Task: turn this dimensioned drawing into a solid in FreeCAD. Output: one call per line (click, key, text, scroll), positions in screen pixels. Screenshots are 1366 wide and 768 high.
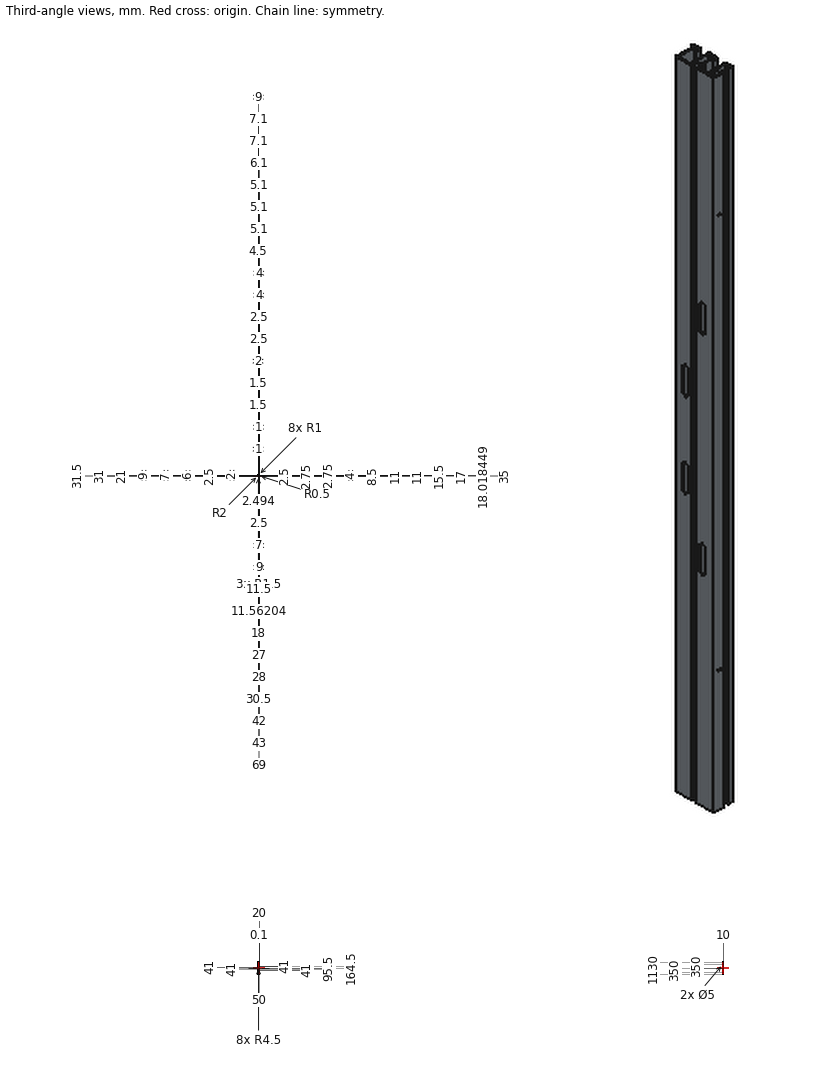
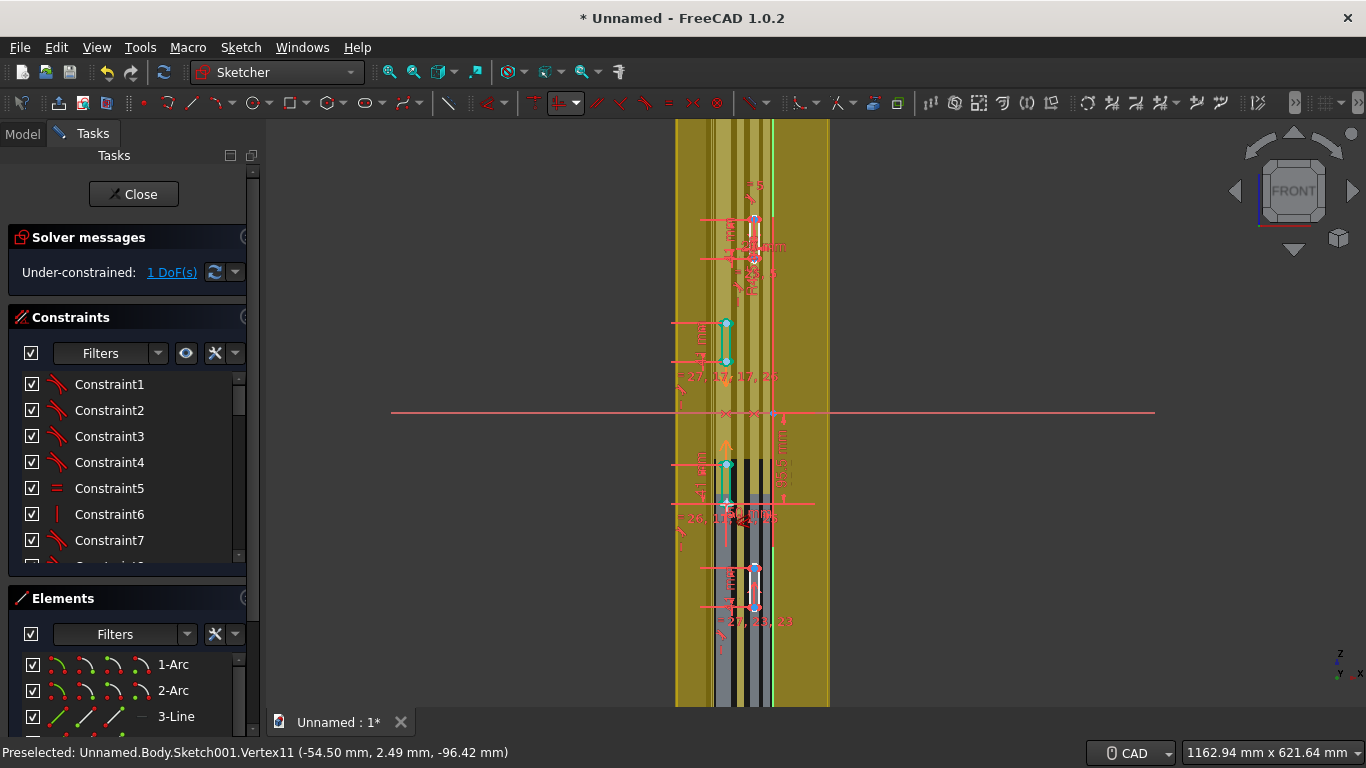
scroll(750, 259, up, 6)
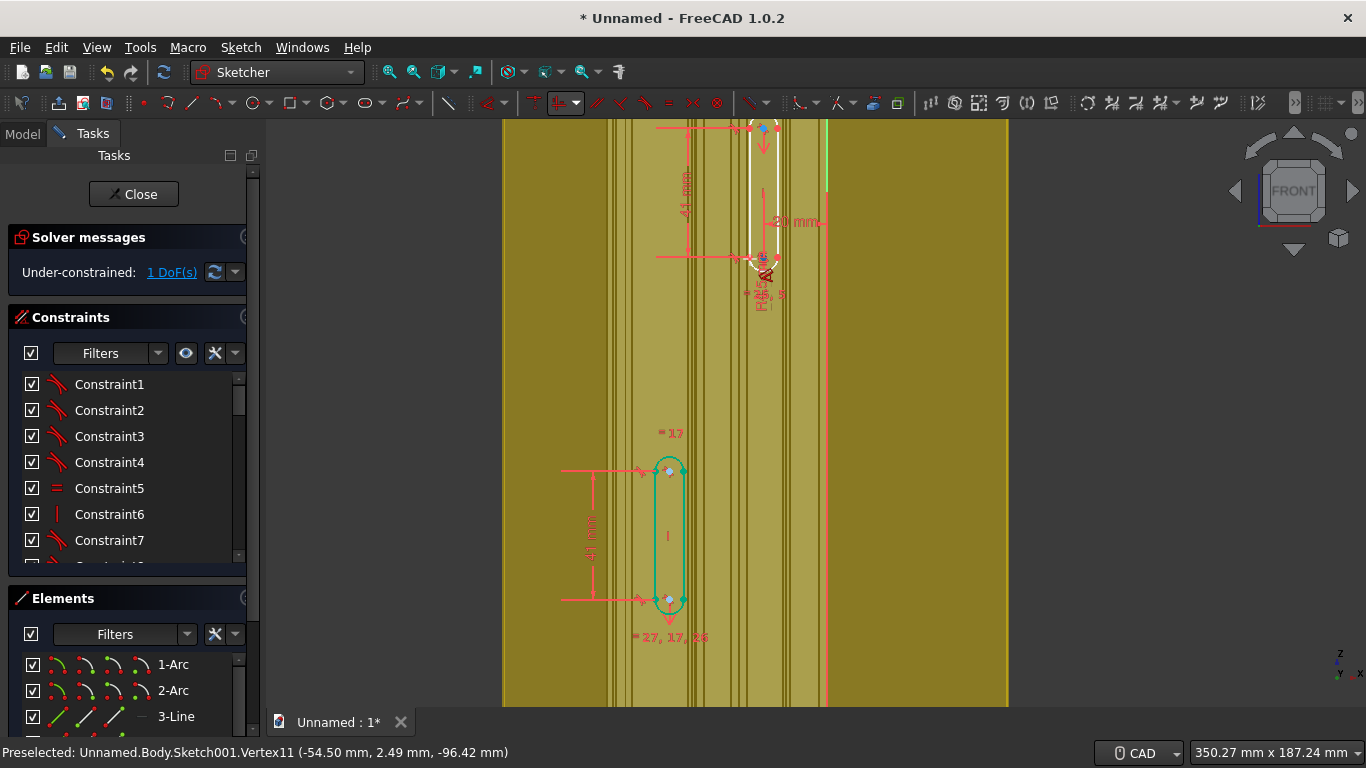
click(750, 257)
click(861, 468)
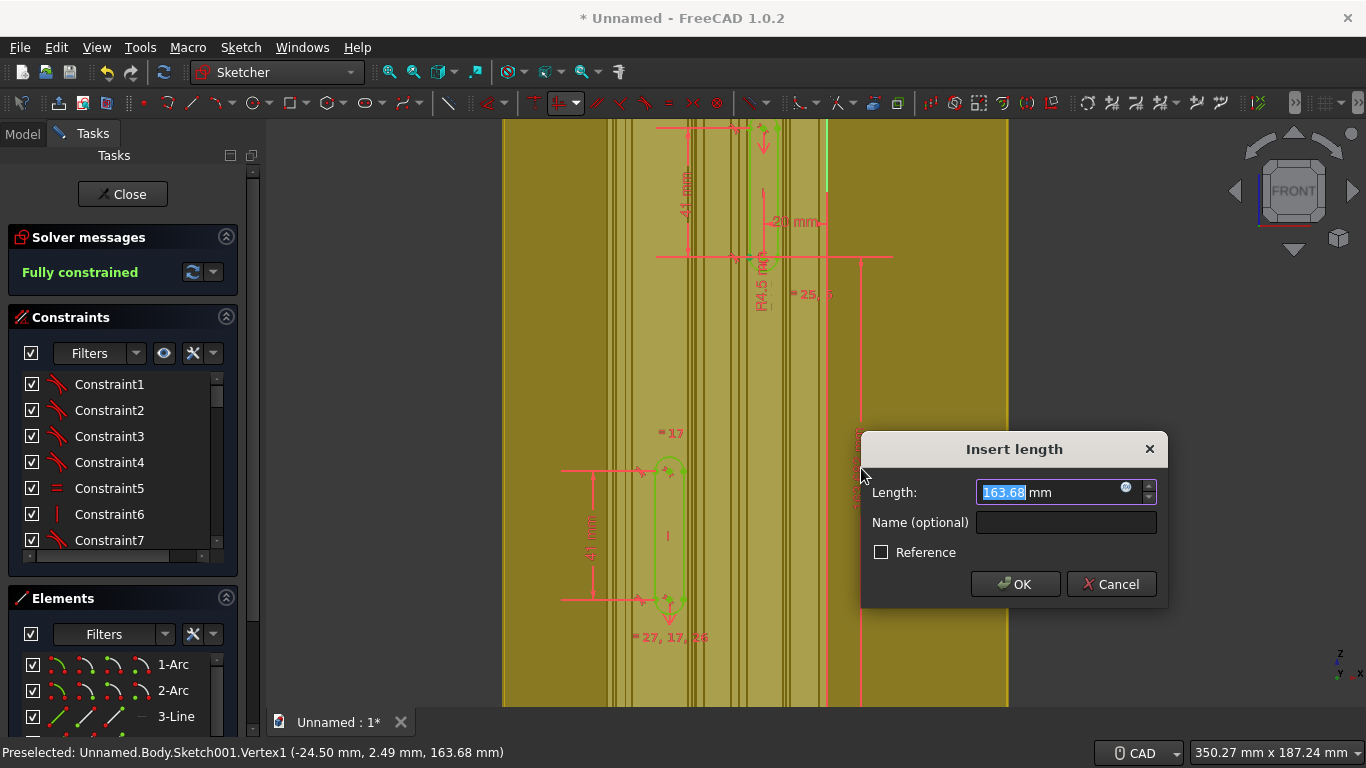
text(164.5)
key(Return)
key(Escape)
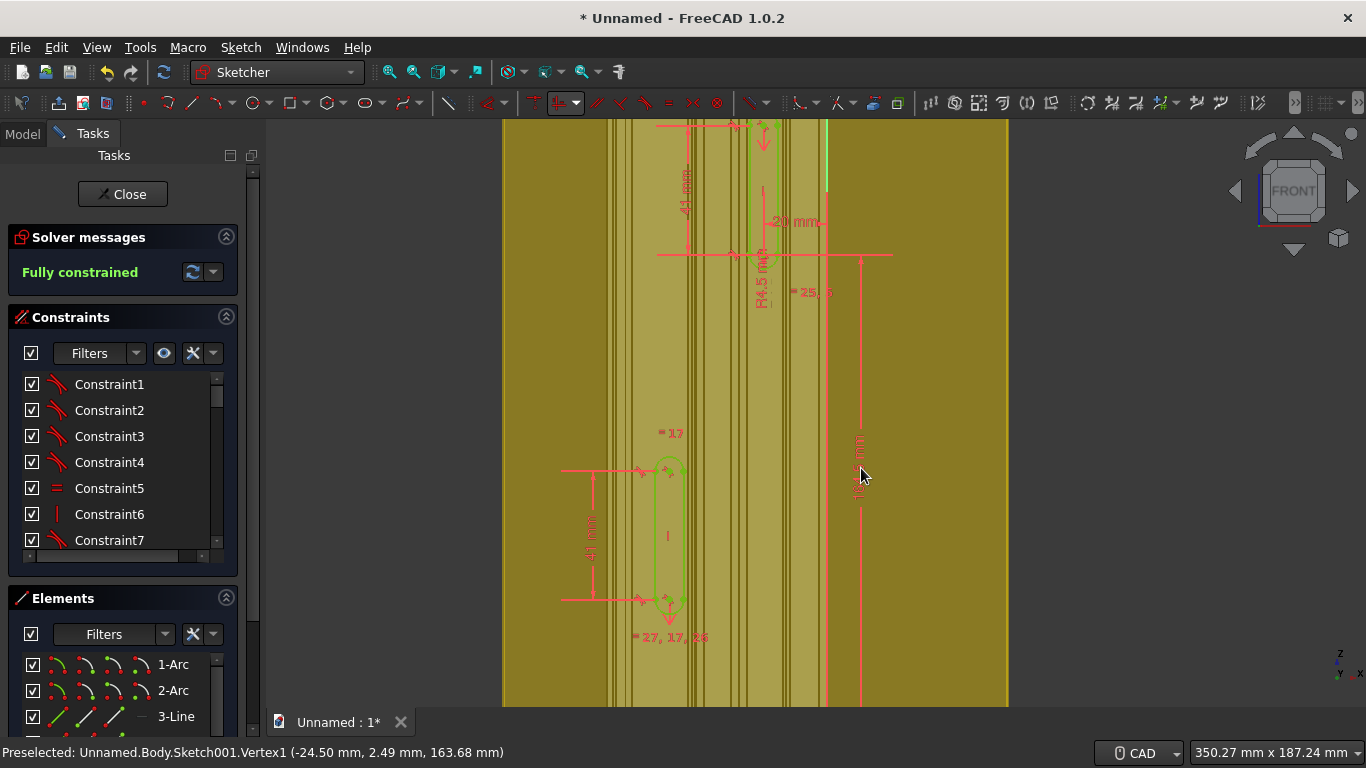
click(123, 194)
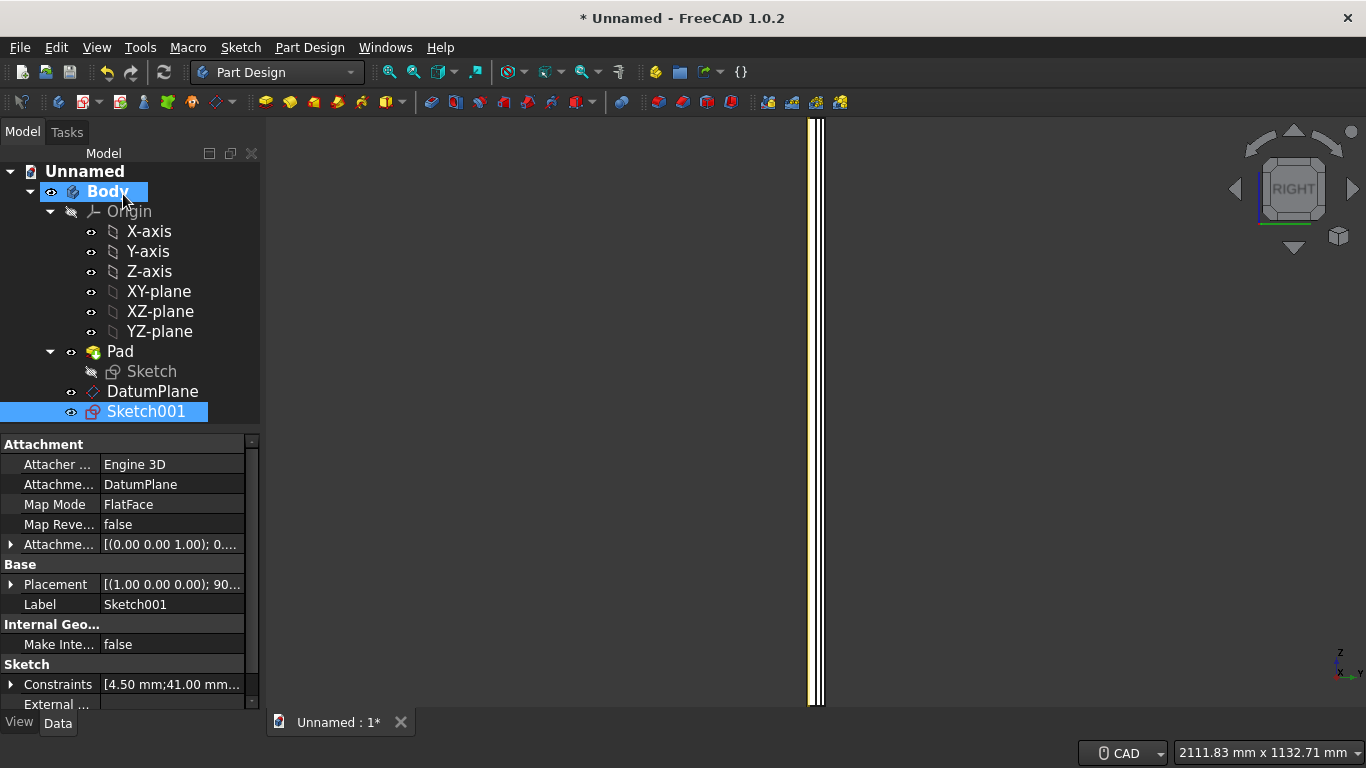
click(432, 102)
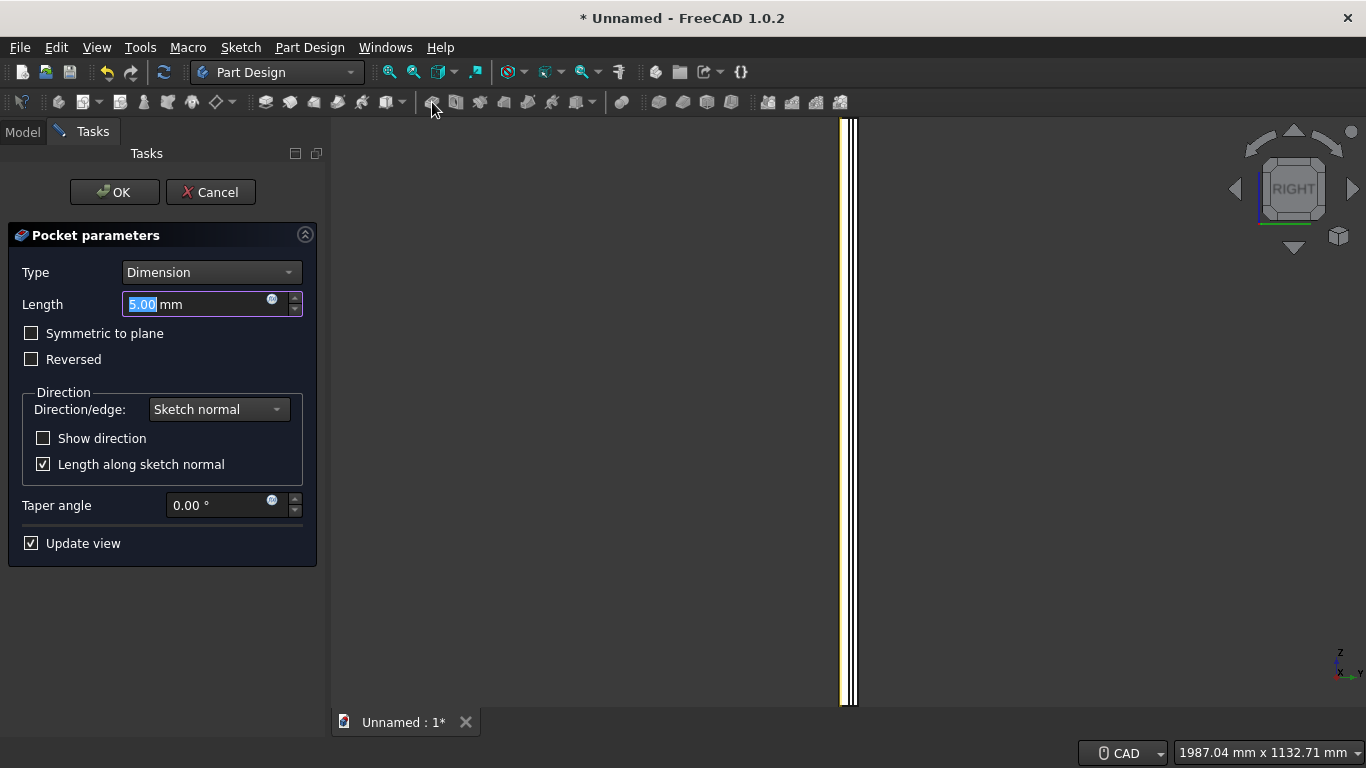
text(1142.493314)
key(Tab)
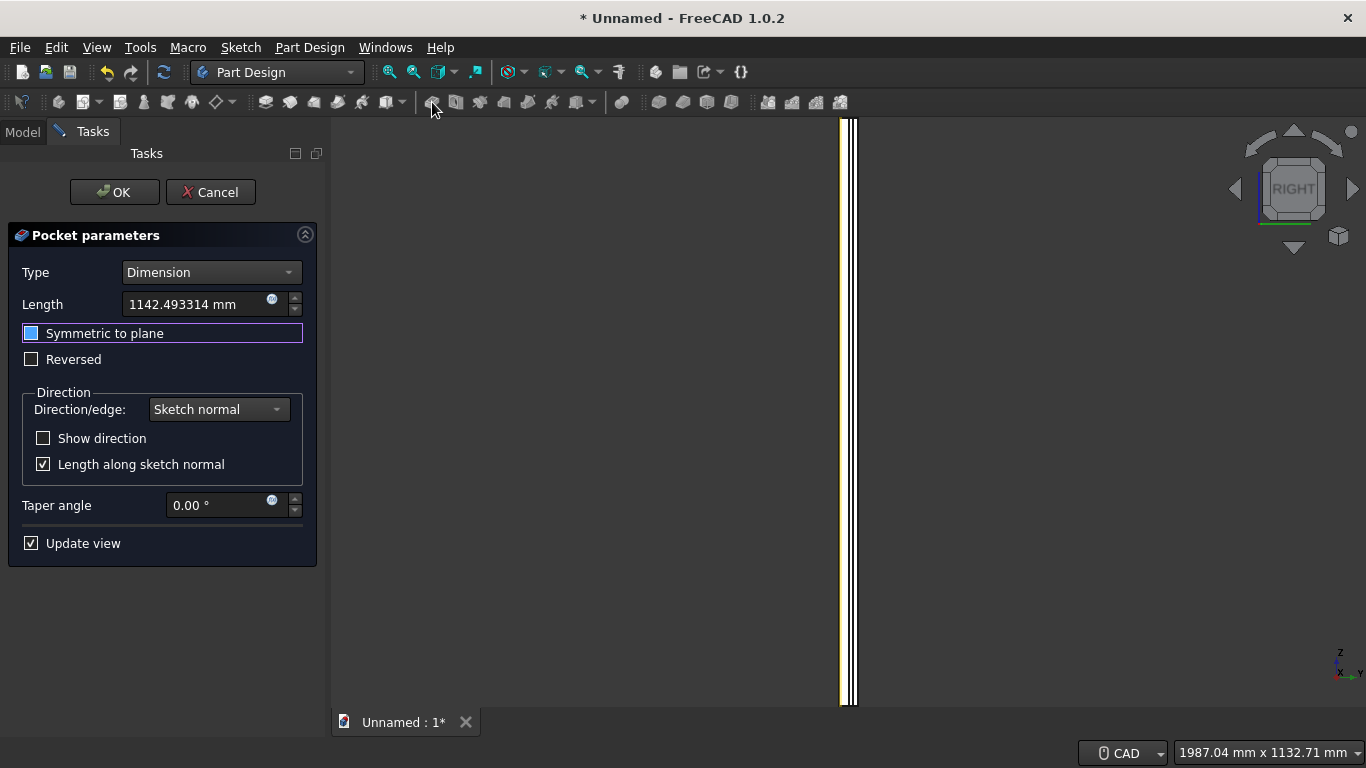
click(30, 333)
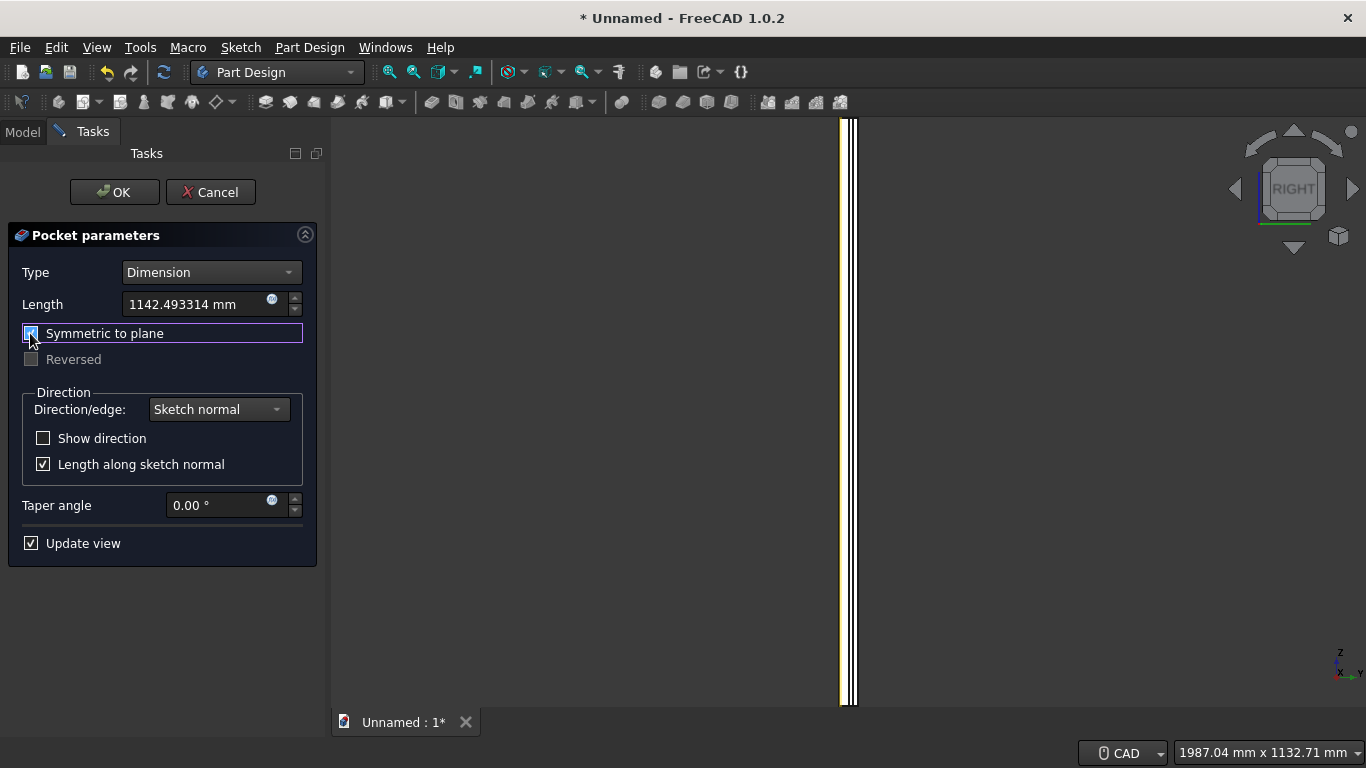
click(115, 192)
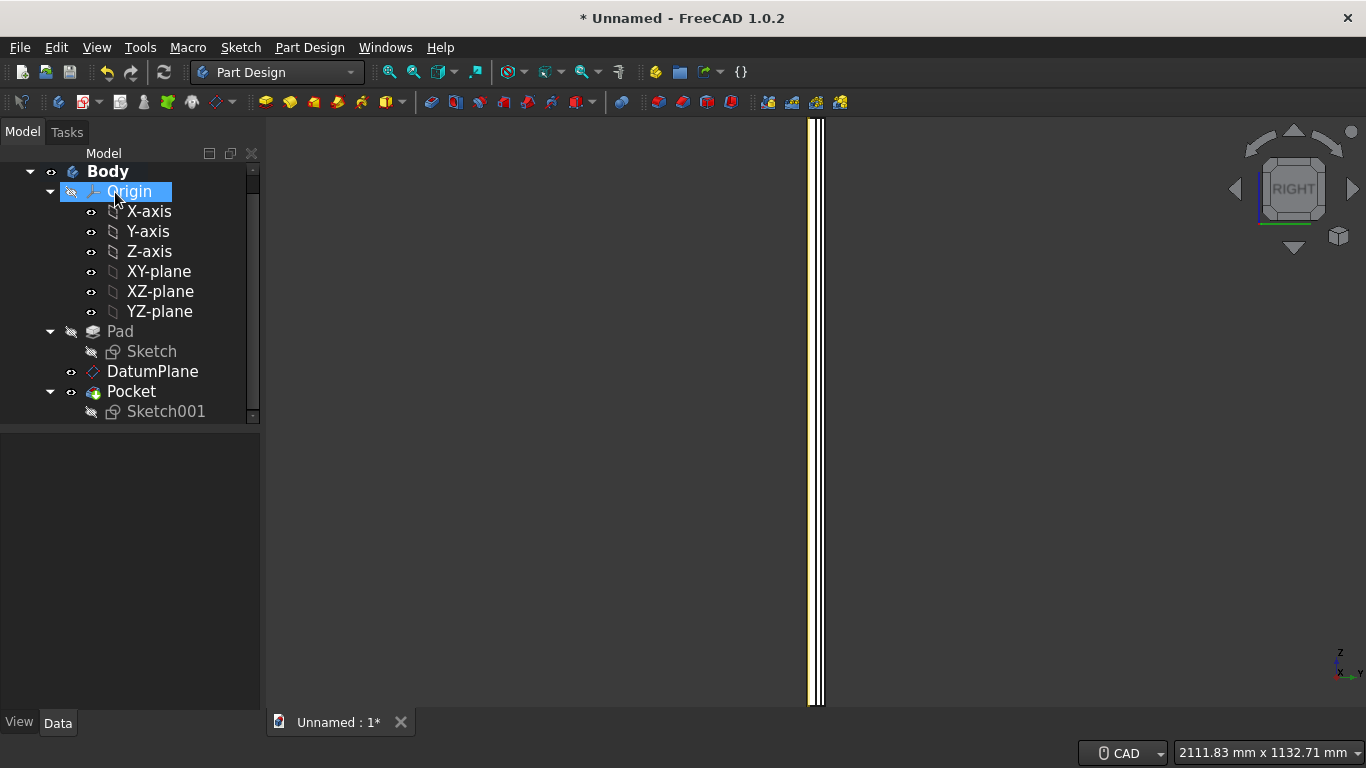
click(116, 372)
key(space)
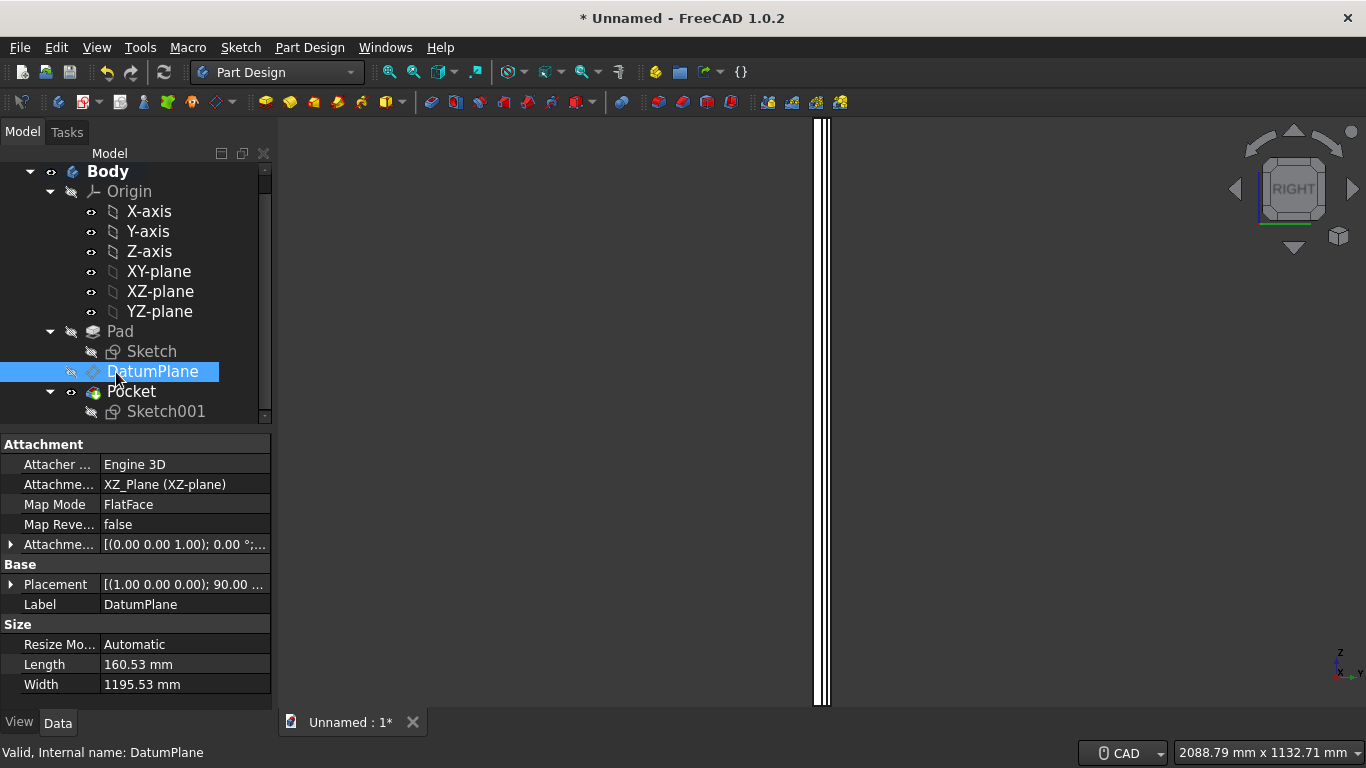
click(318, 667)